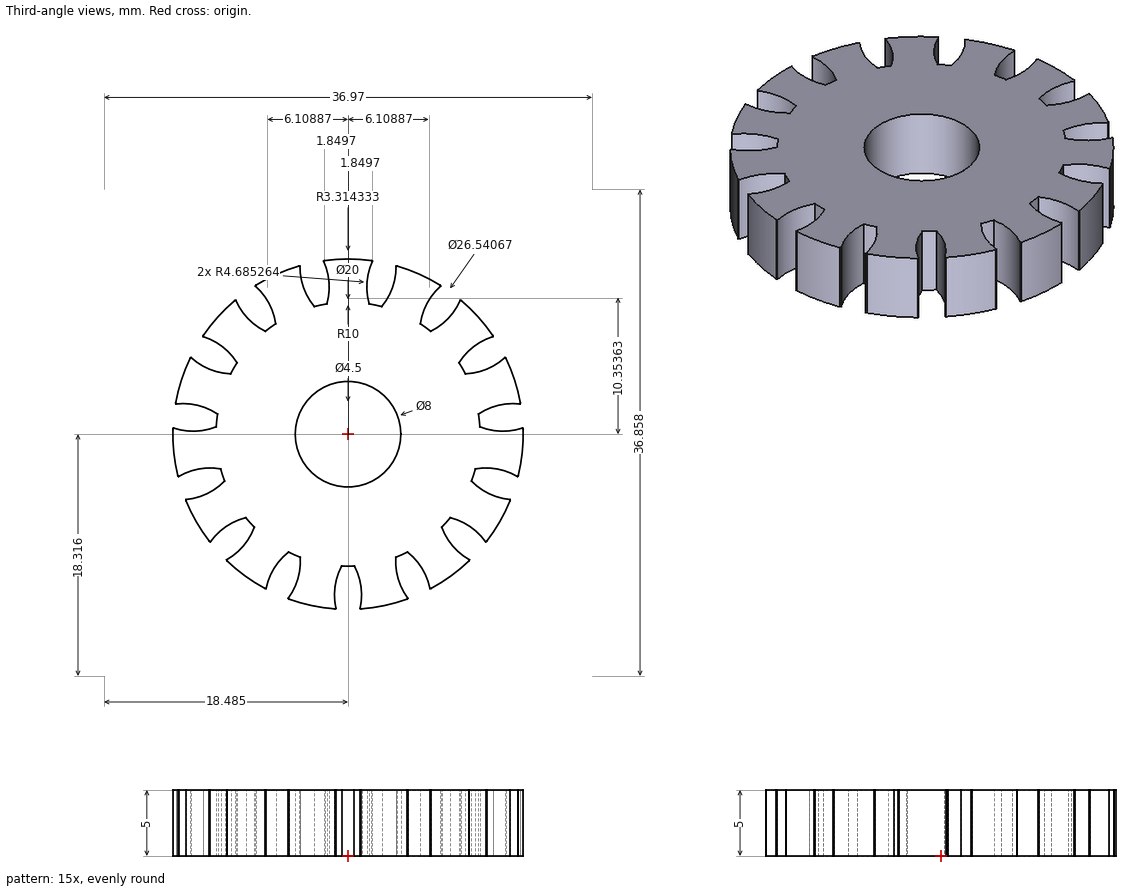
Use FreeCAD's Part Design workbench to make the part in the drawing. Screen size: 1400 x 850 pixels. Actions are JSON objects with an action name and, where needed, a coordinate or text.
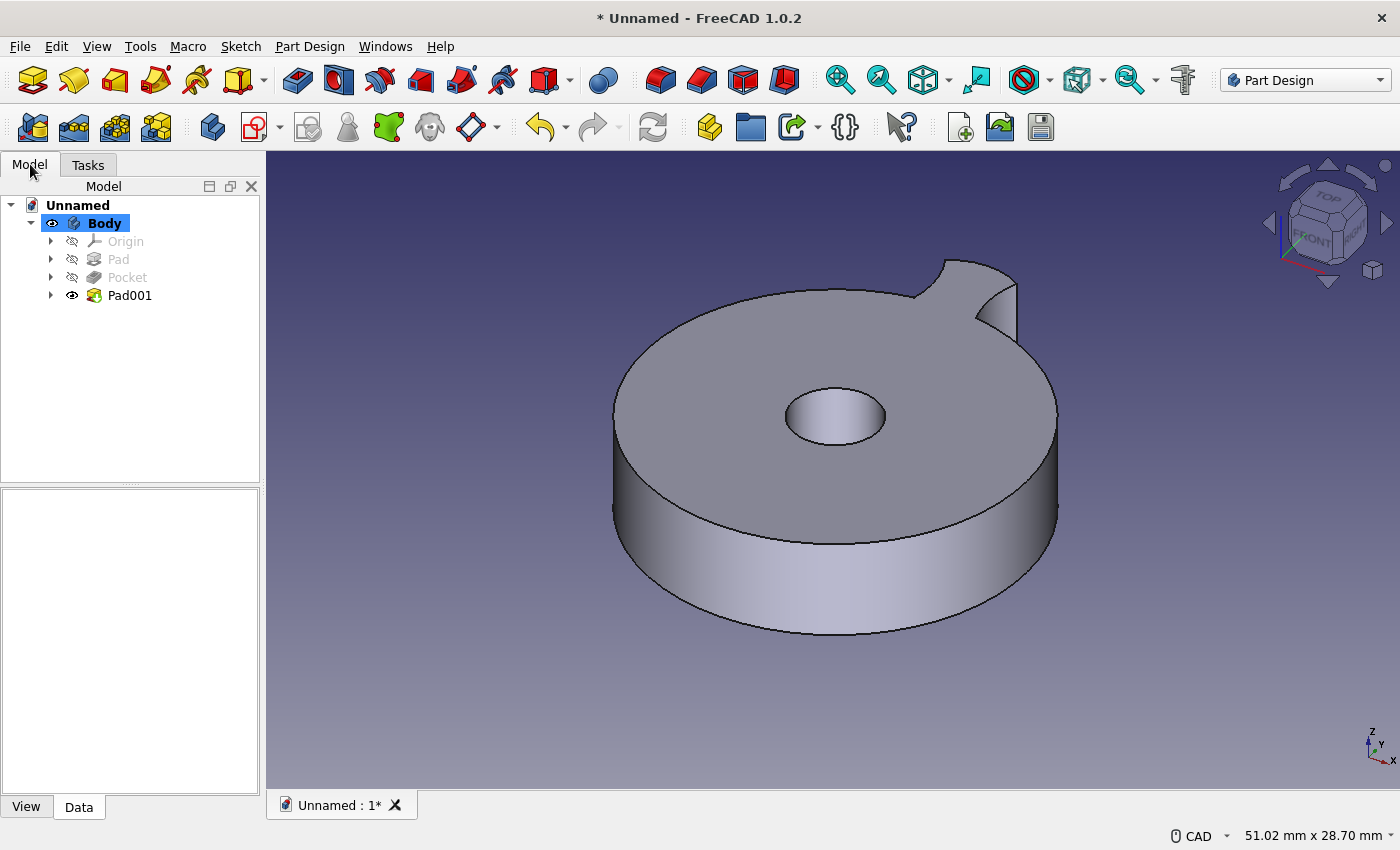
{"action": "left_click", "coordinate": [117, 295]}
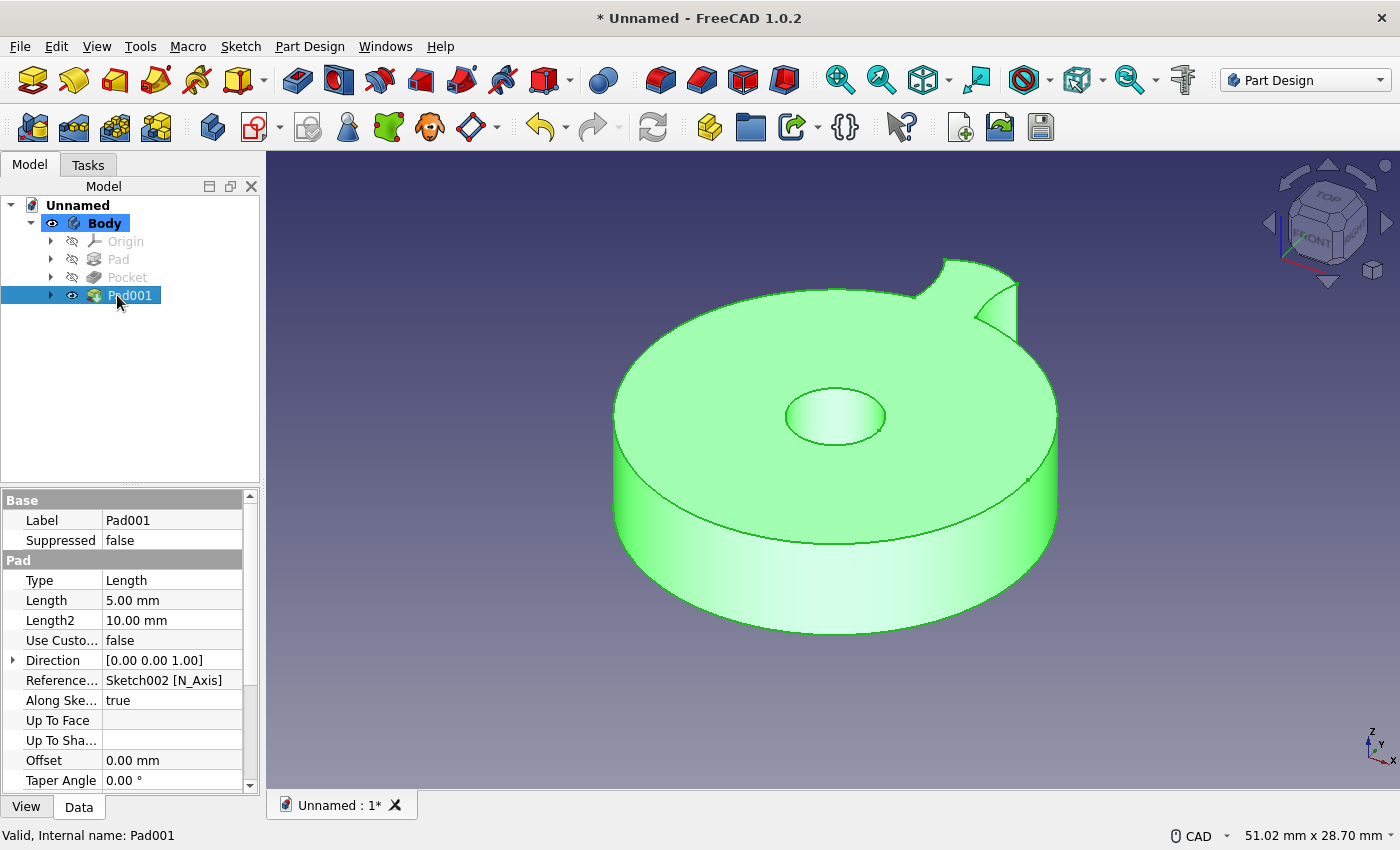
{"action": "left_click", "coordinate": [115, 128]}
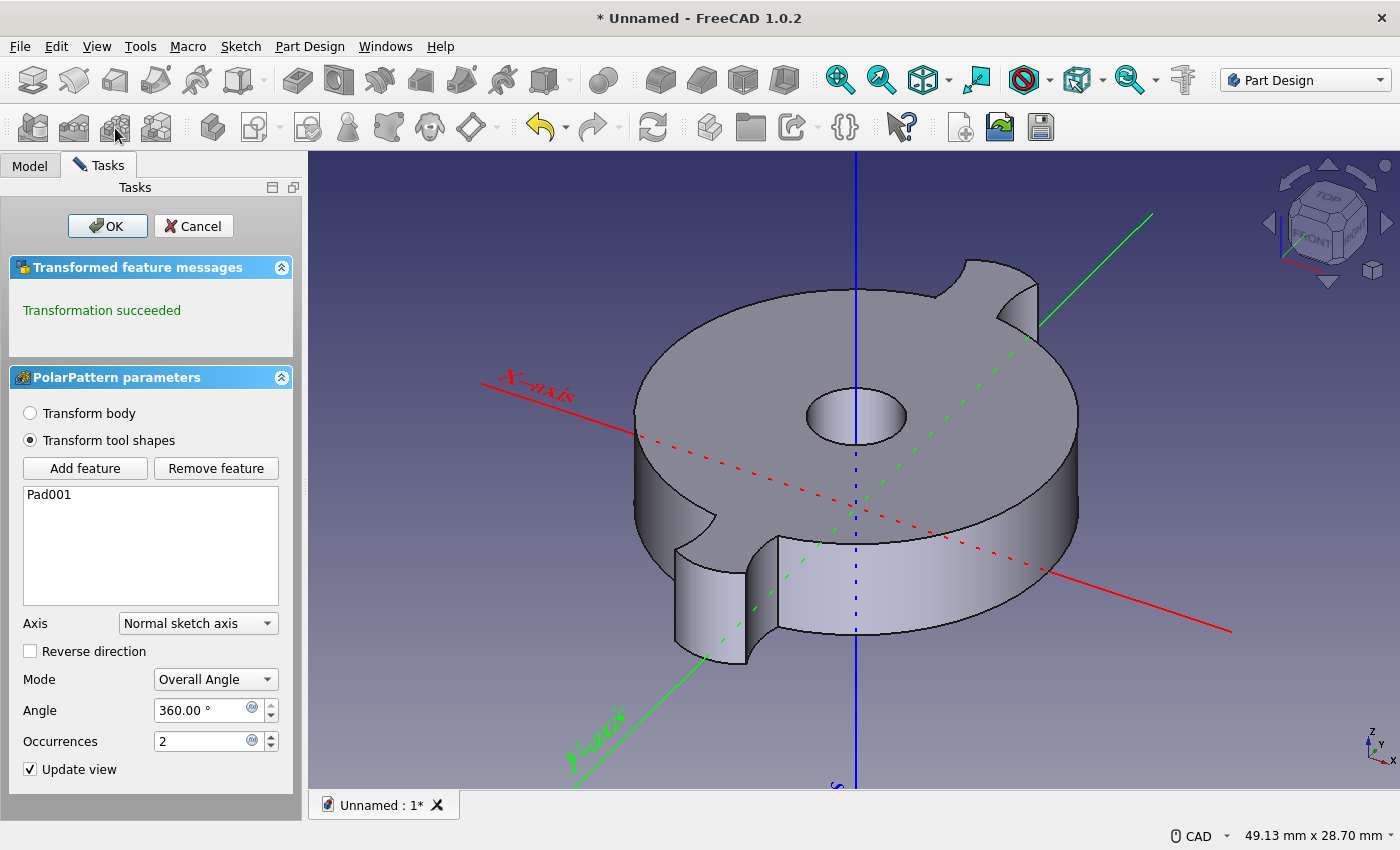
{"action": "left_click", "coordinate": [199, 624]}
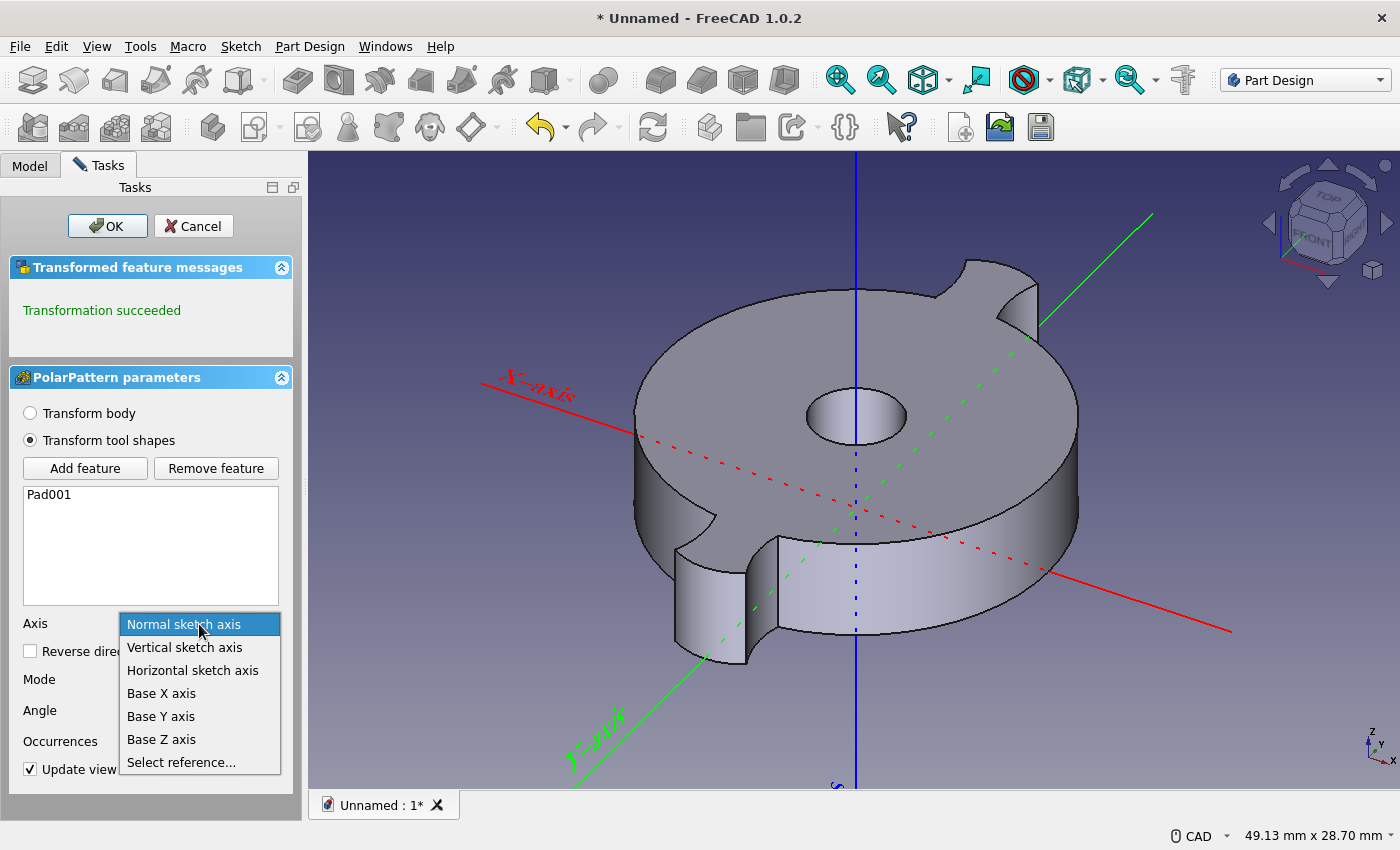
{"action": "left_click", "coordinate": [198, 740]}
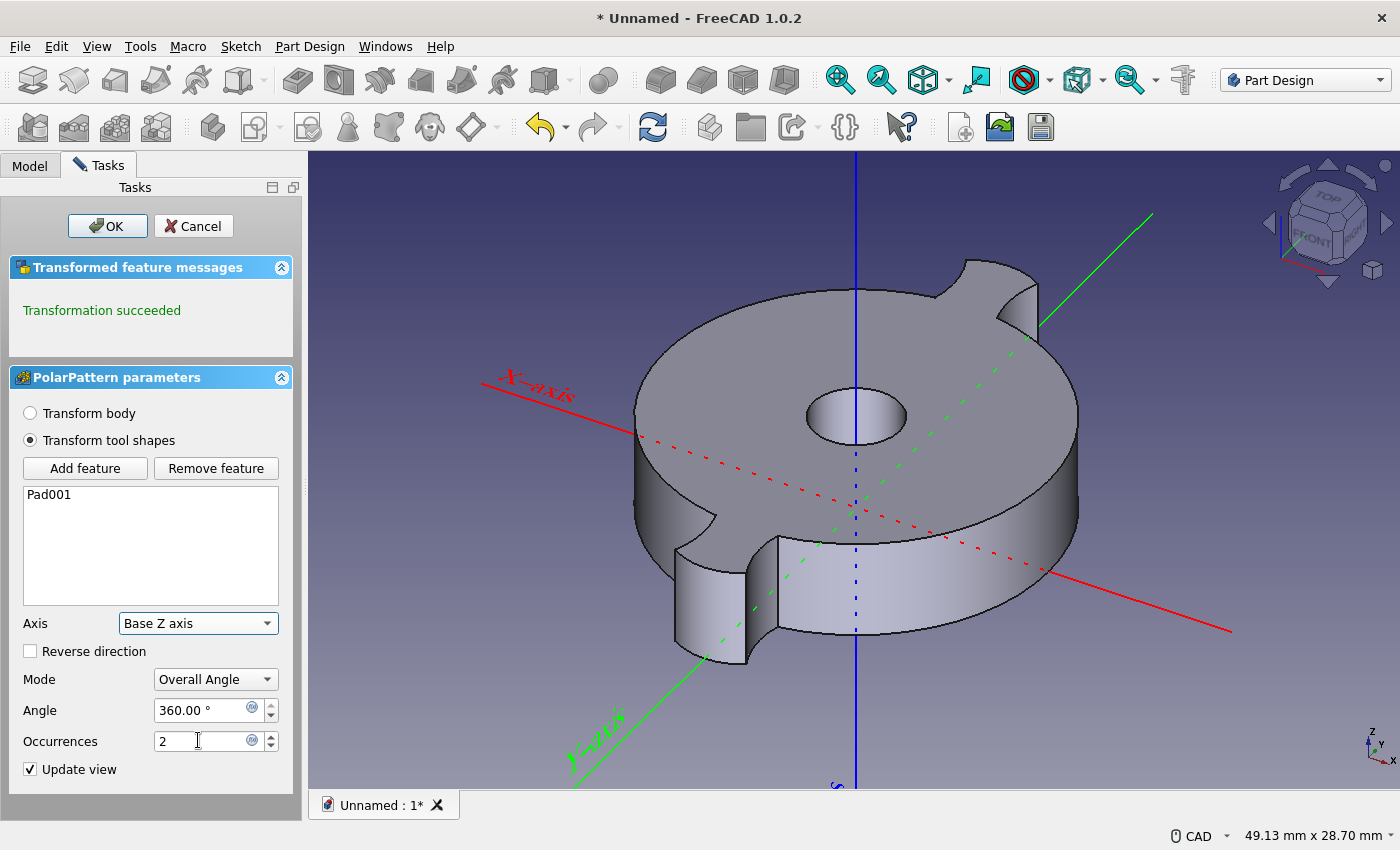
{"action": "triple_click", "coordinate": [210, 742]}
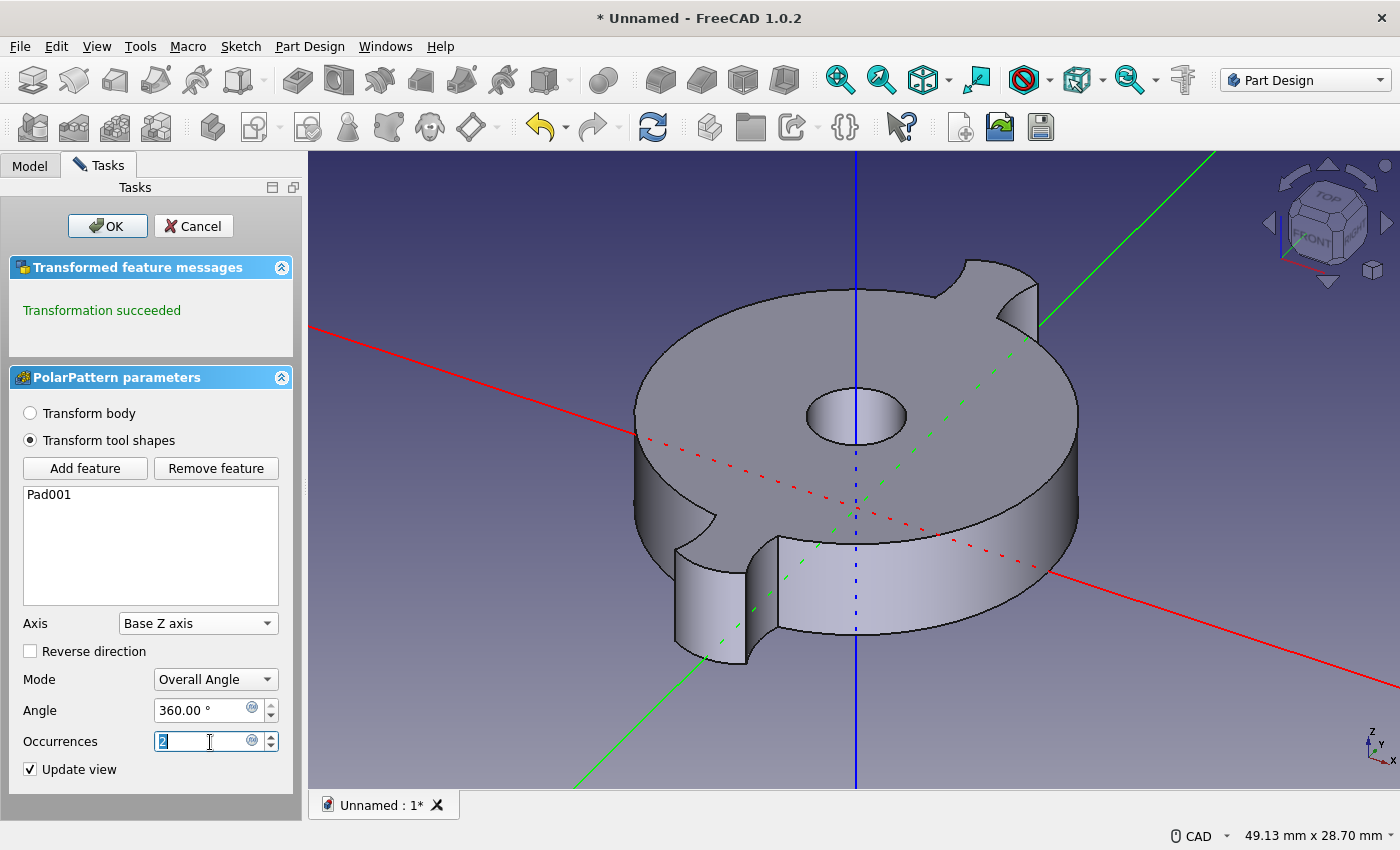
{"action": "type", "text": "15"}
{"action": "key", "text": "Tab"}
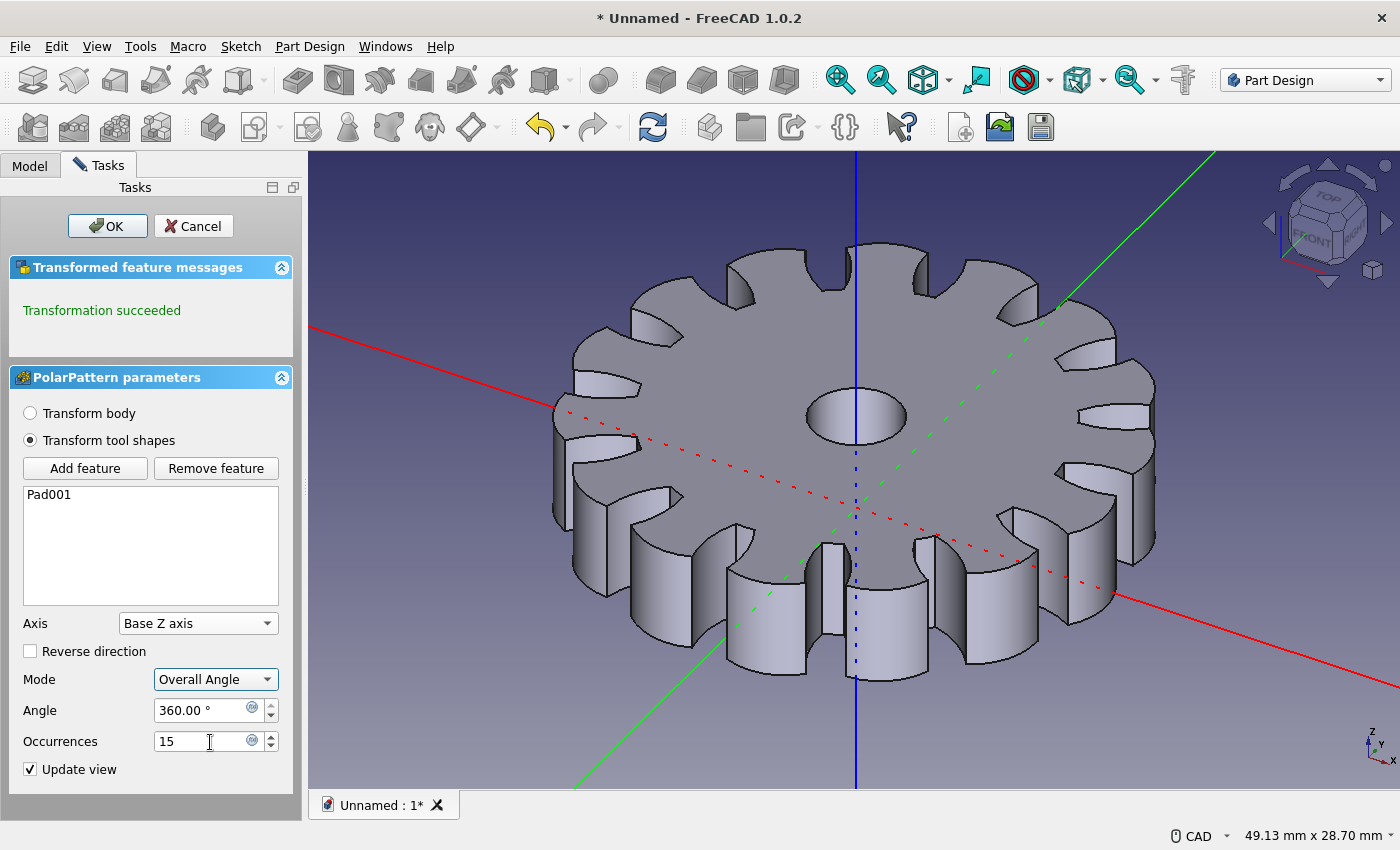
{"action": "left_click", "coordinate": [108, 226]}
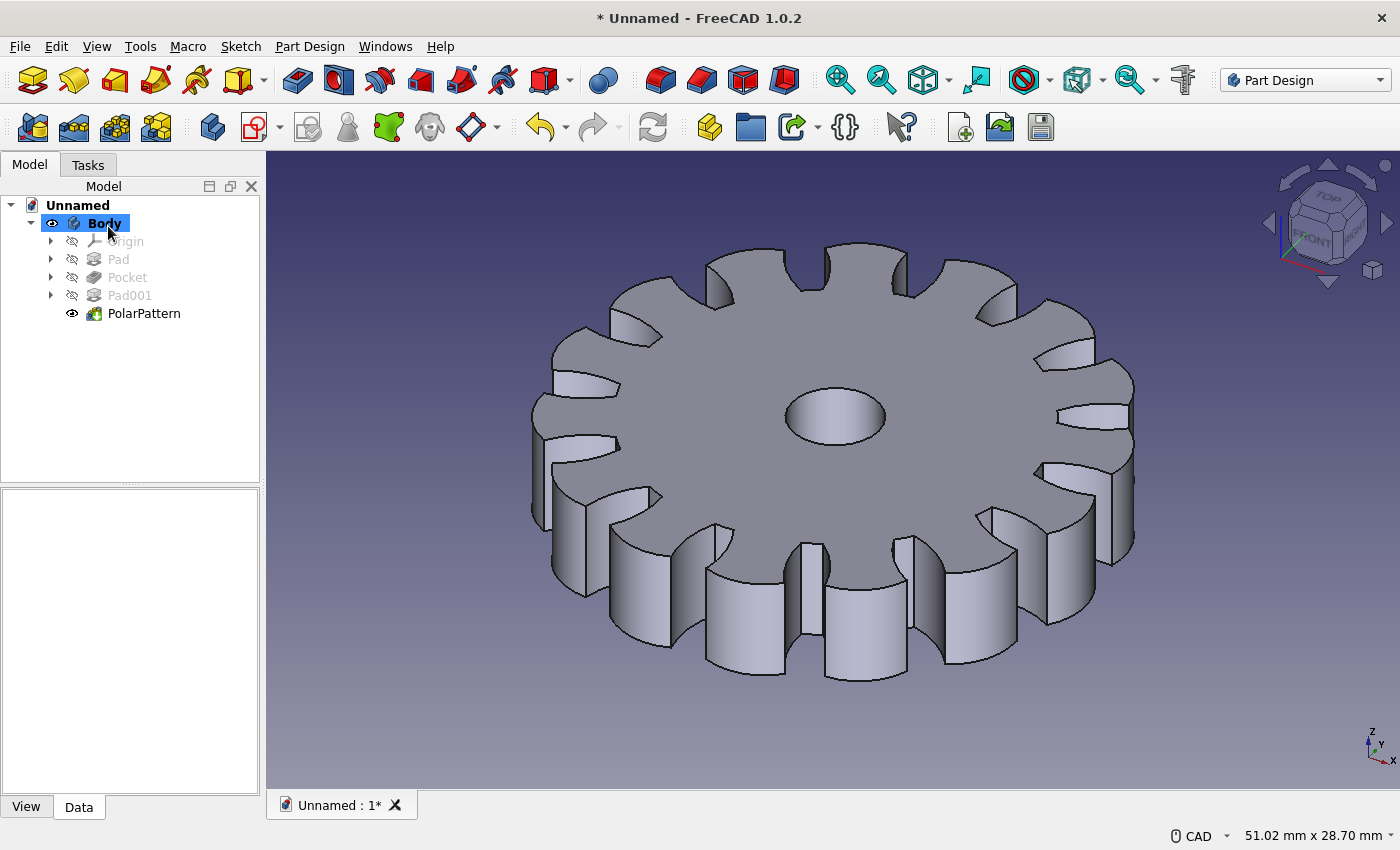
{"action": "key", "text": "5"}